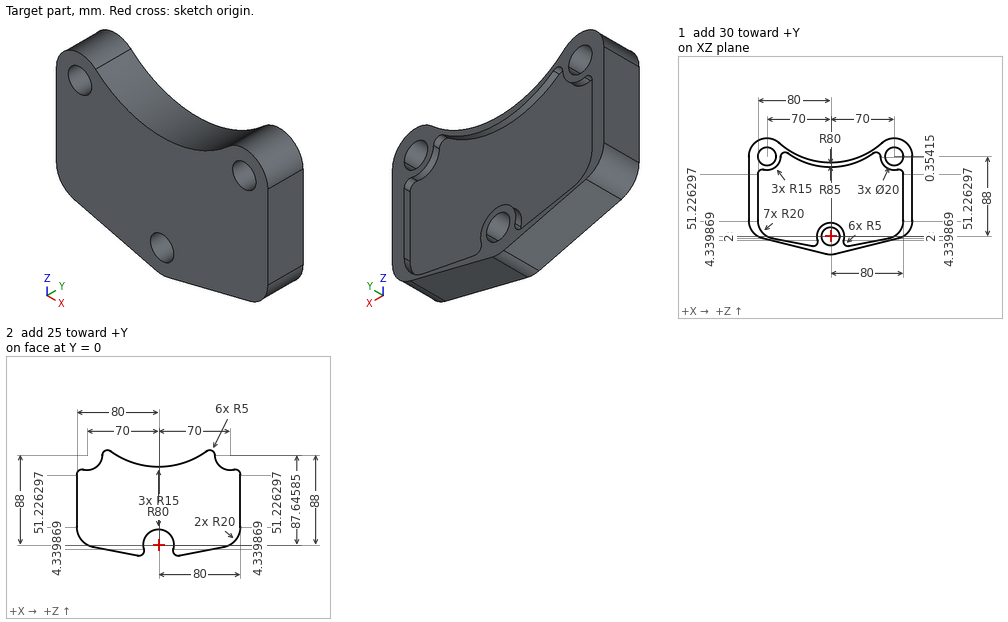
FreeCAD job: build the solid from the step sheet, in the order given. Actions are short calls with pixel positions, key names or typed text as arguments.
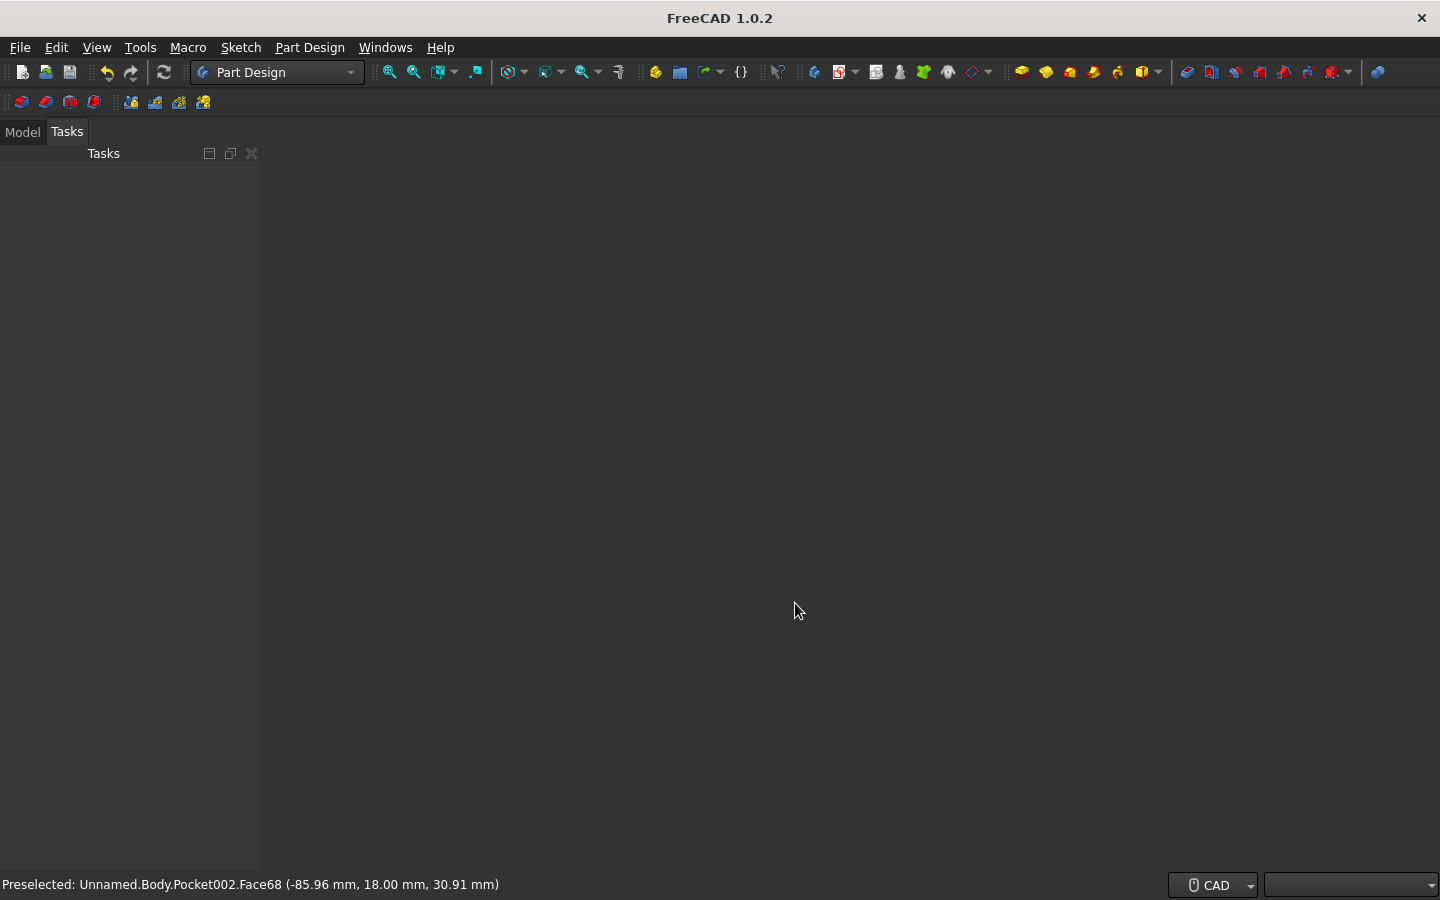
click(22, 72)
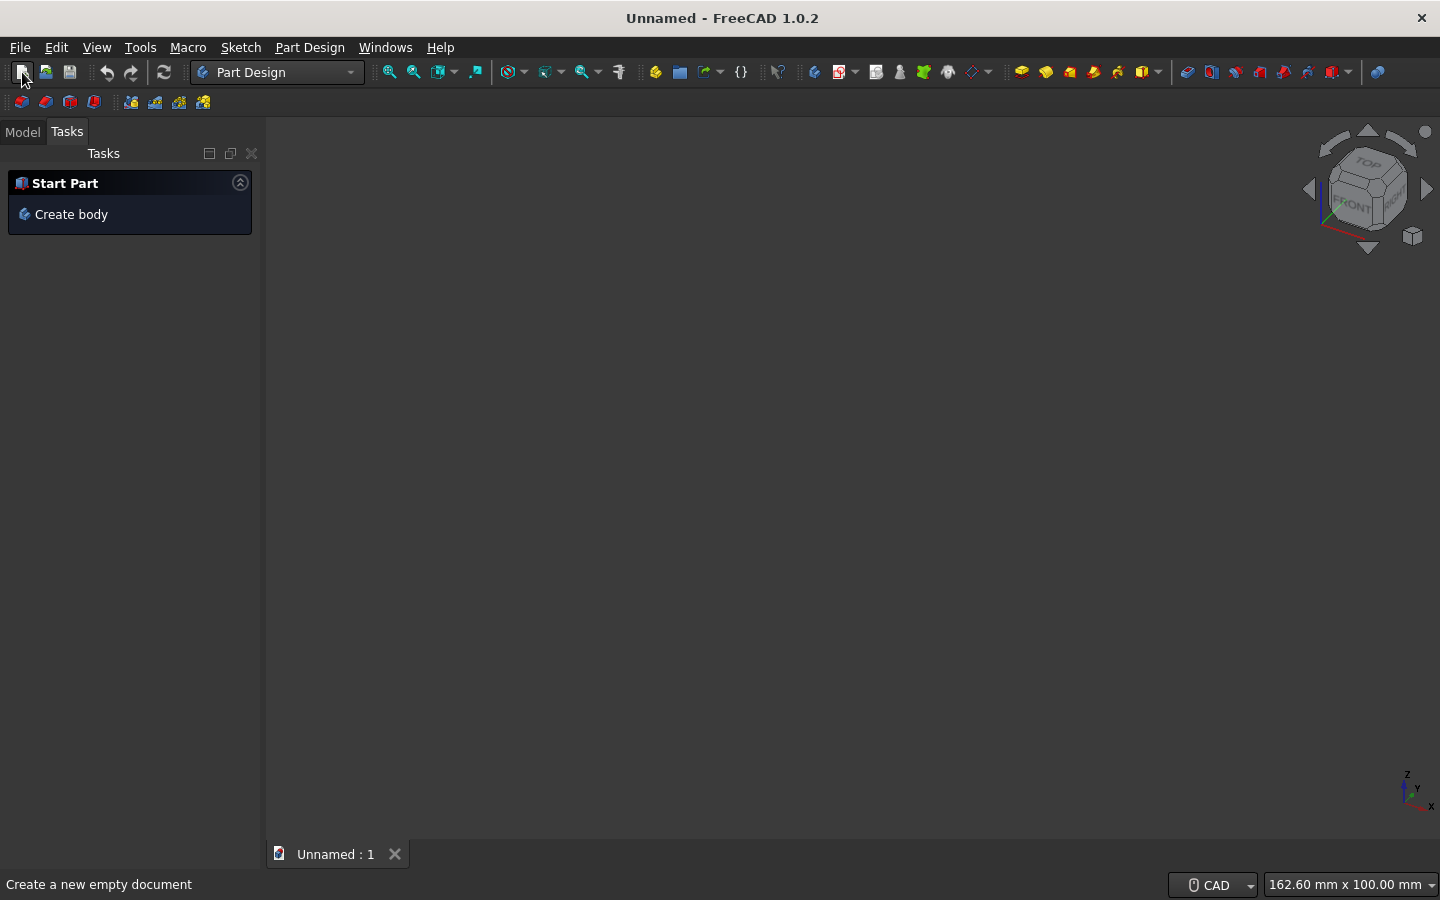
click(840, 72)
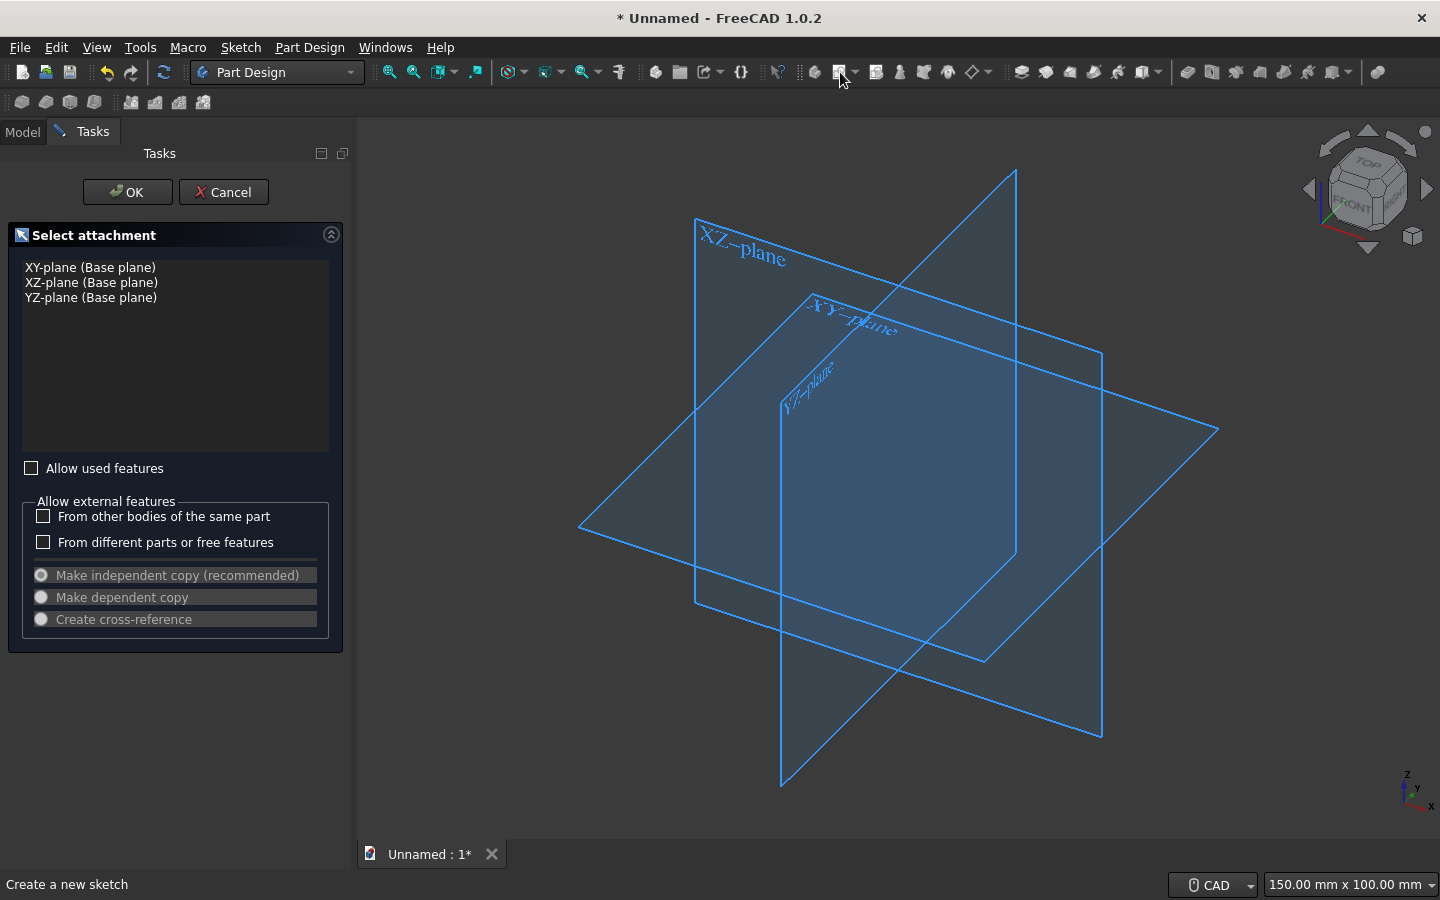
click(82, 282)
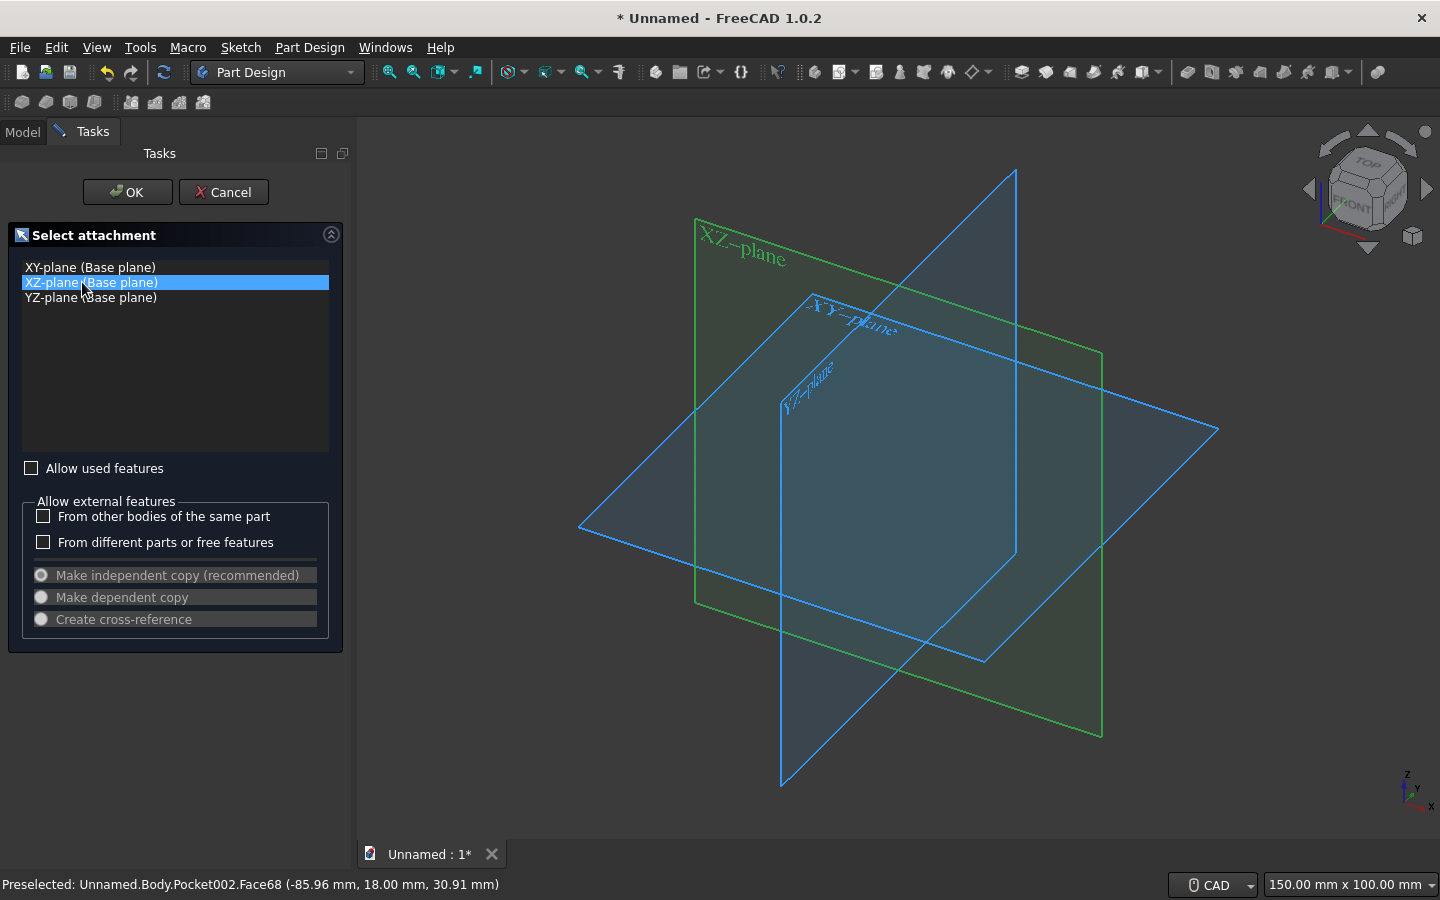
click(128, 192)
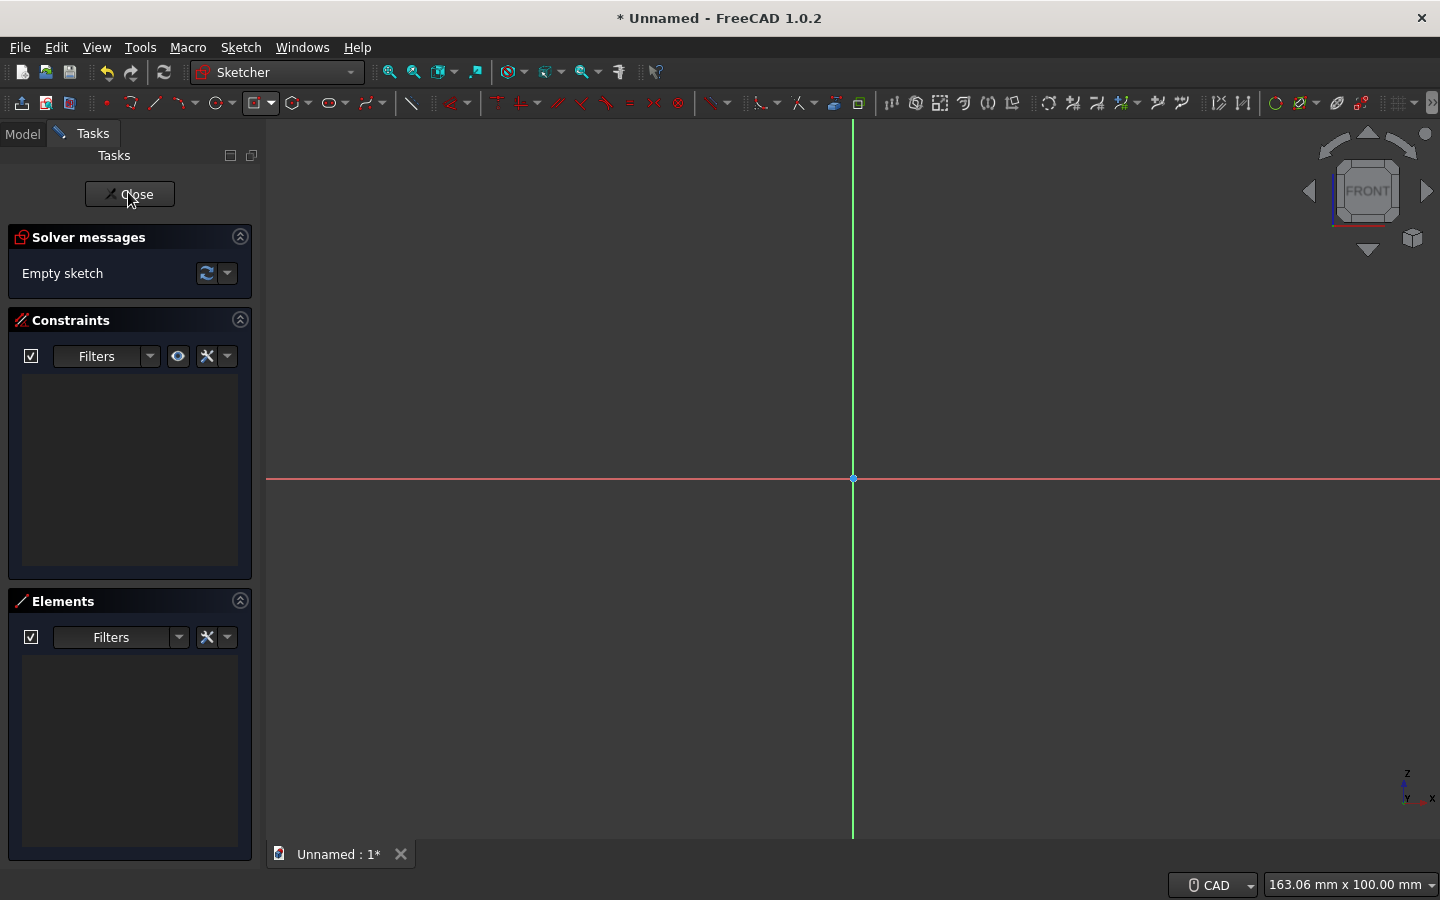
scroll(701, 811, down, 3)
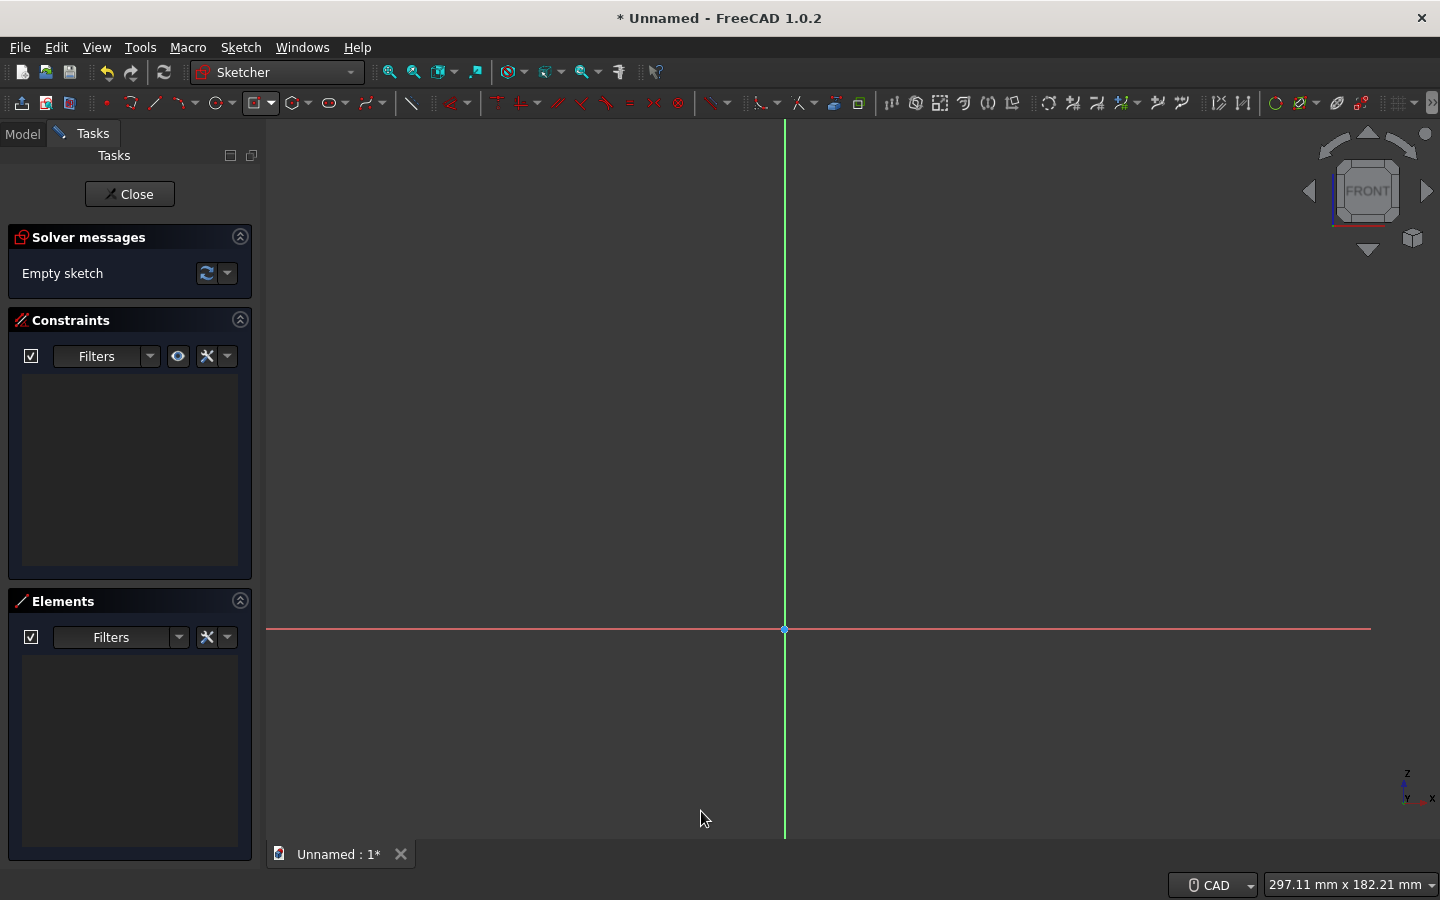
click(156, 104)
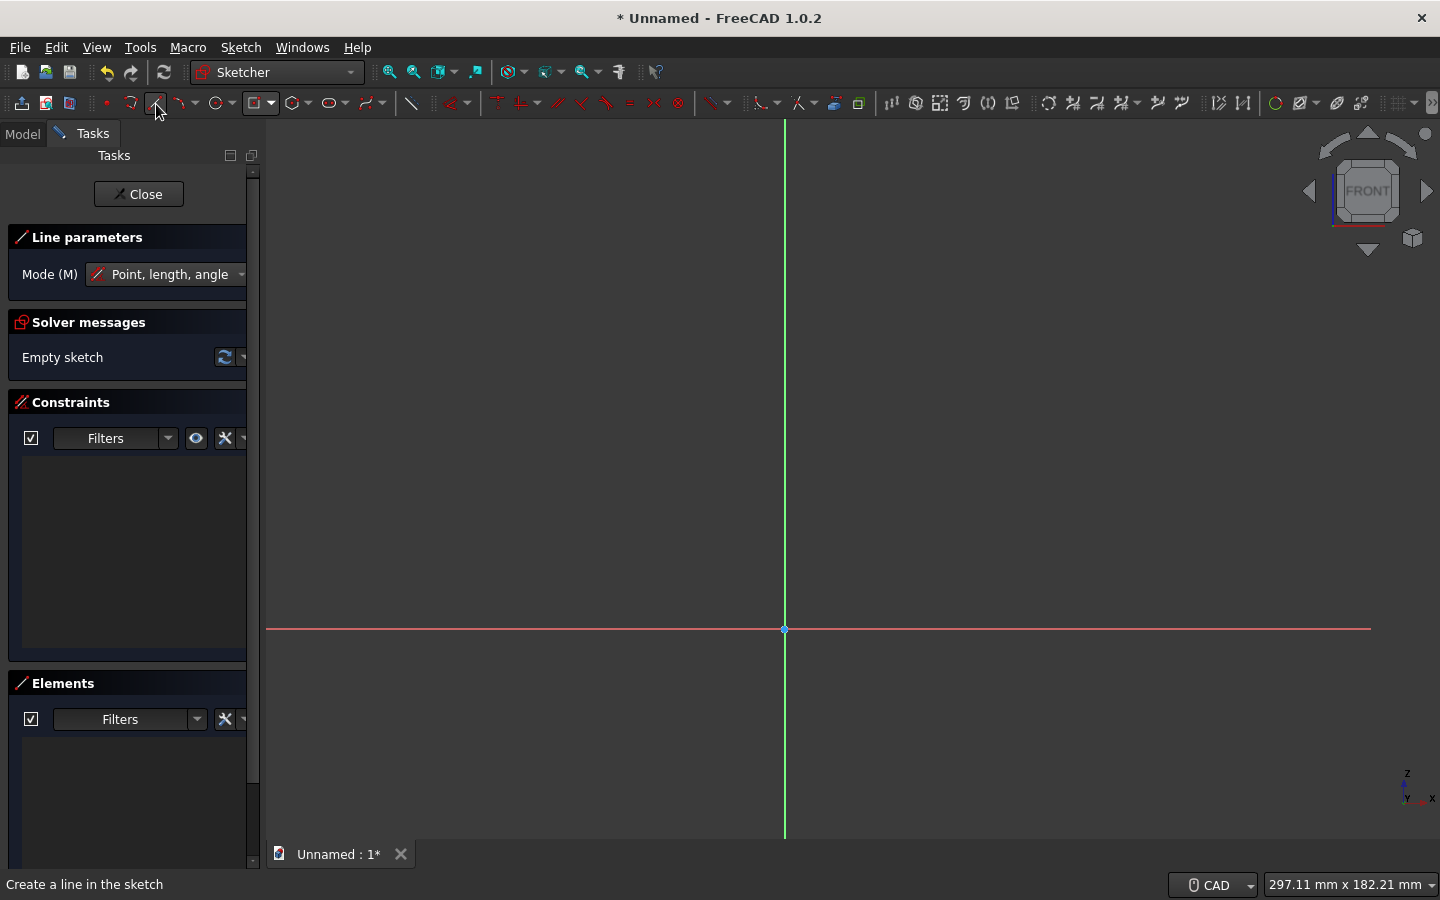
click(429, 560)
click(429, 282)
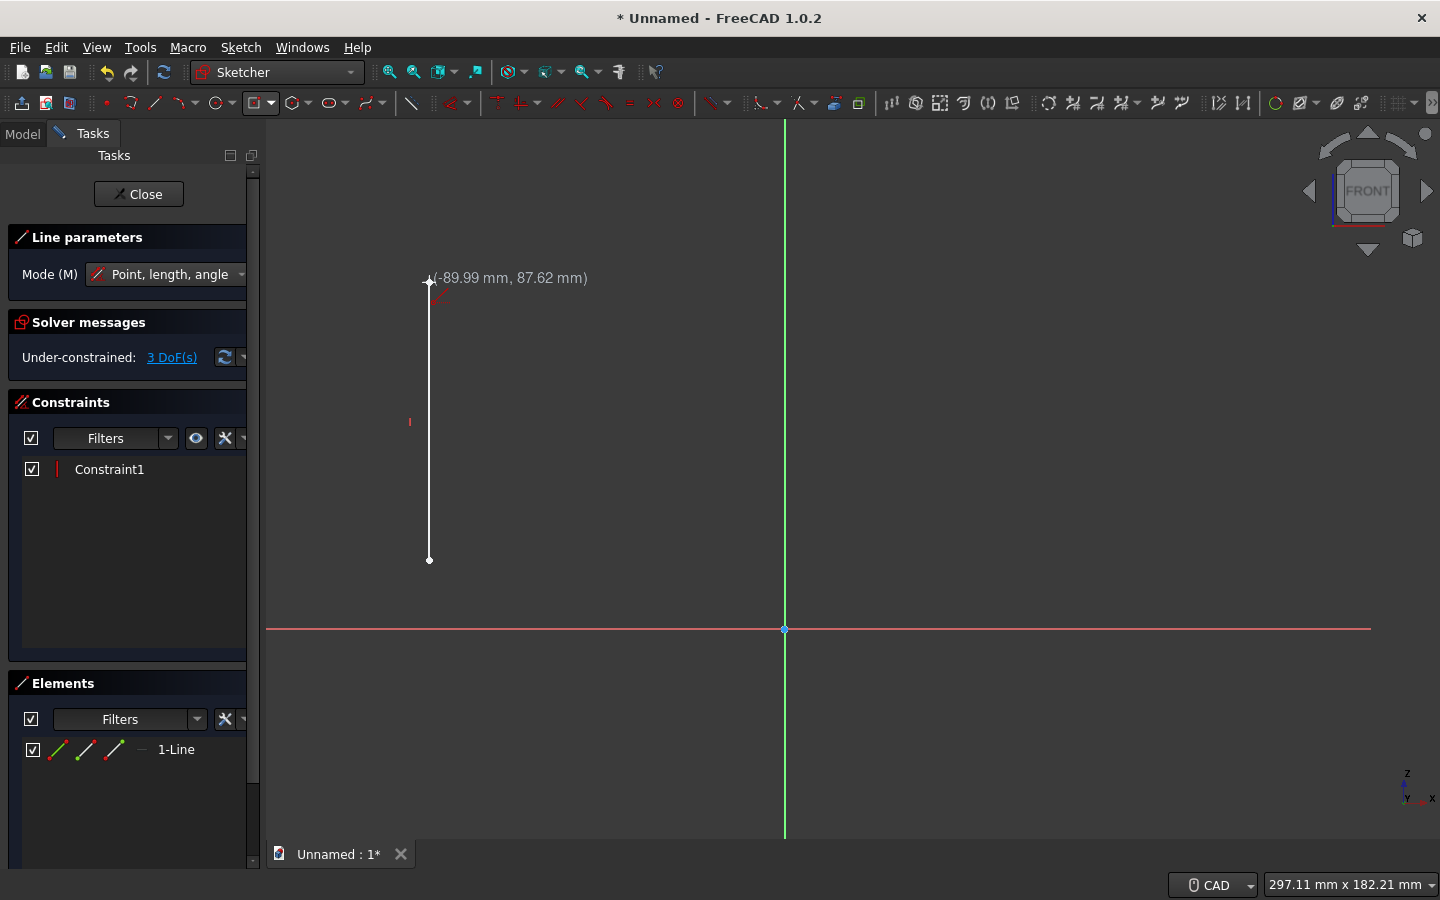
click(1140, 282)
click(1140, 560)